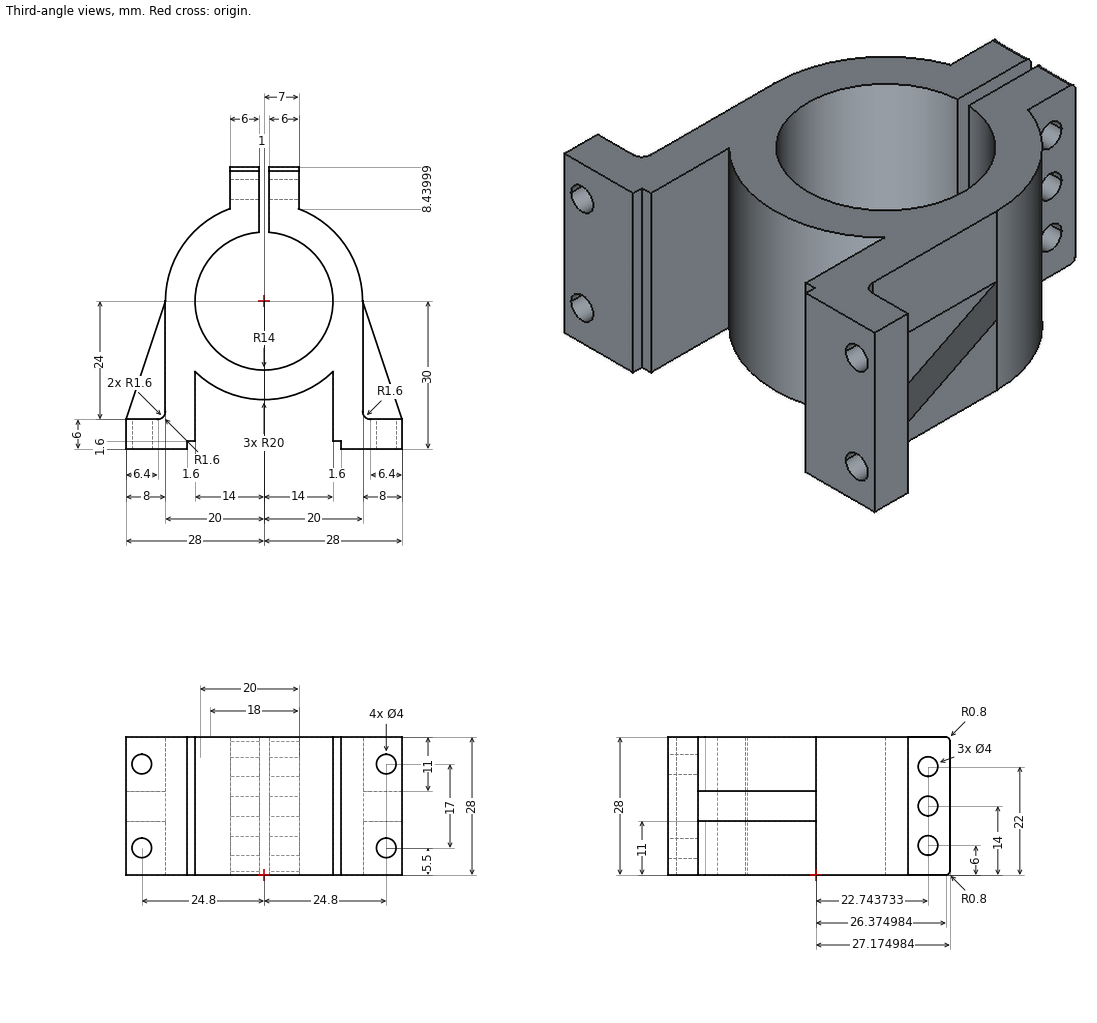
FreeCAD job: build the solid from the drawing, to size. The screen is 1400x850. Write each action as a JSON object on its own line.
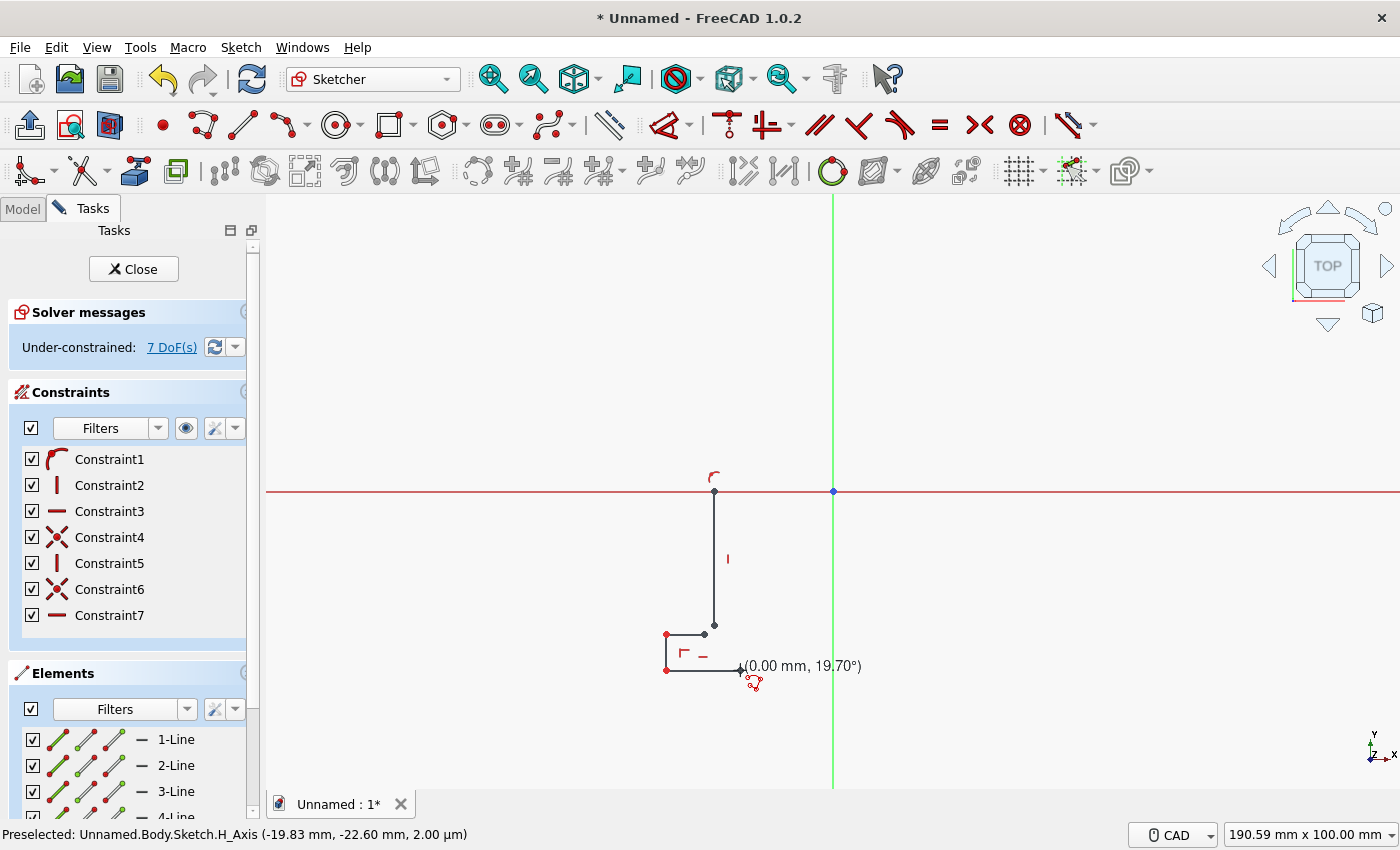
{"action": "scroll", "coordinate": [740, 660], "scroll_direction": "up", "scroll_amount": 3}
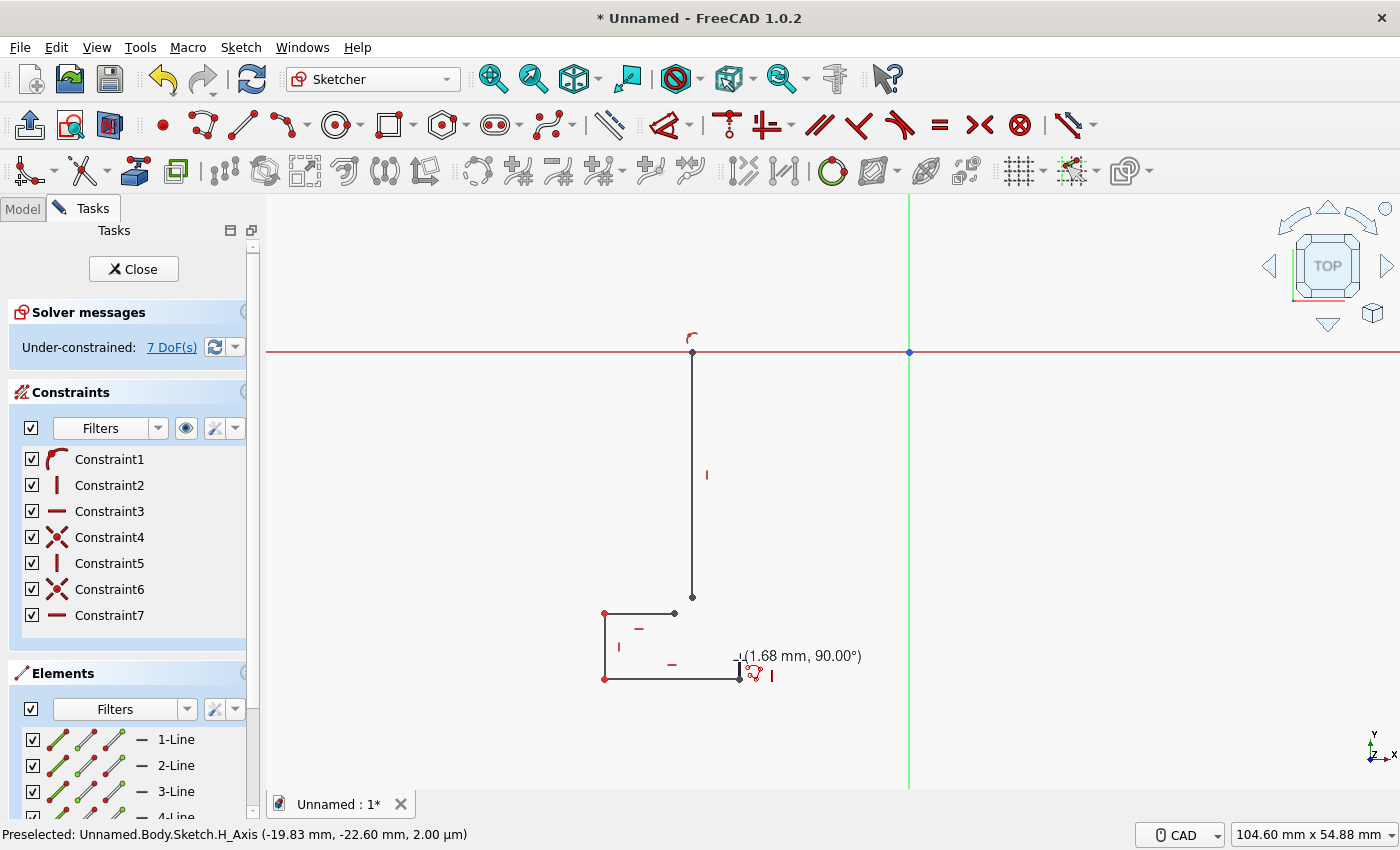
{"action": "left_click", "coordinate": [740, 660]}
{"action": "left_click", "coordinate": [757, 660]}
{"action": "left_click", "coordinate": [757, 507]}
{"action": "right_click", "coordinate": [757, 507]}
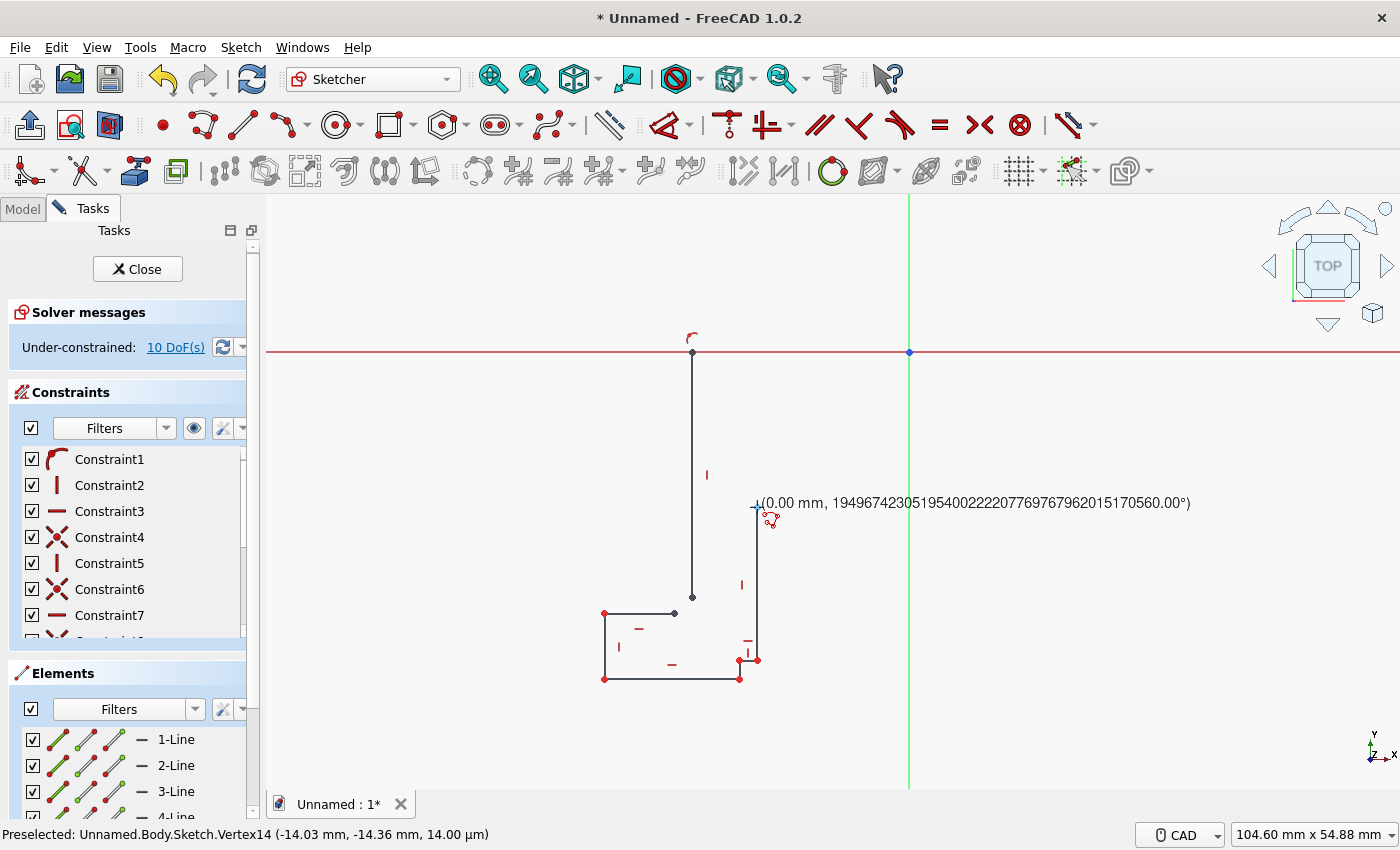
{"action": "left_click", "coordinate": [1061, 507]}
{"action": "left_click", "coordinate": [1061, 660]}
{"action": "left_click", "coordinate": [1078, 660]}
{"action": "left_click", "coordinate": [1078, 678]}
{"action": "left_click", "coordinate": [1213, 678]}
{"action": "left_click", "coordinate": [1213, 613]}
{"action": "left_click", "coordinate": [1143, 613]}
{"action": "right_click", "coordinate": [1143, 613]}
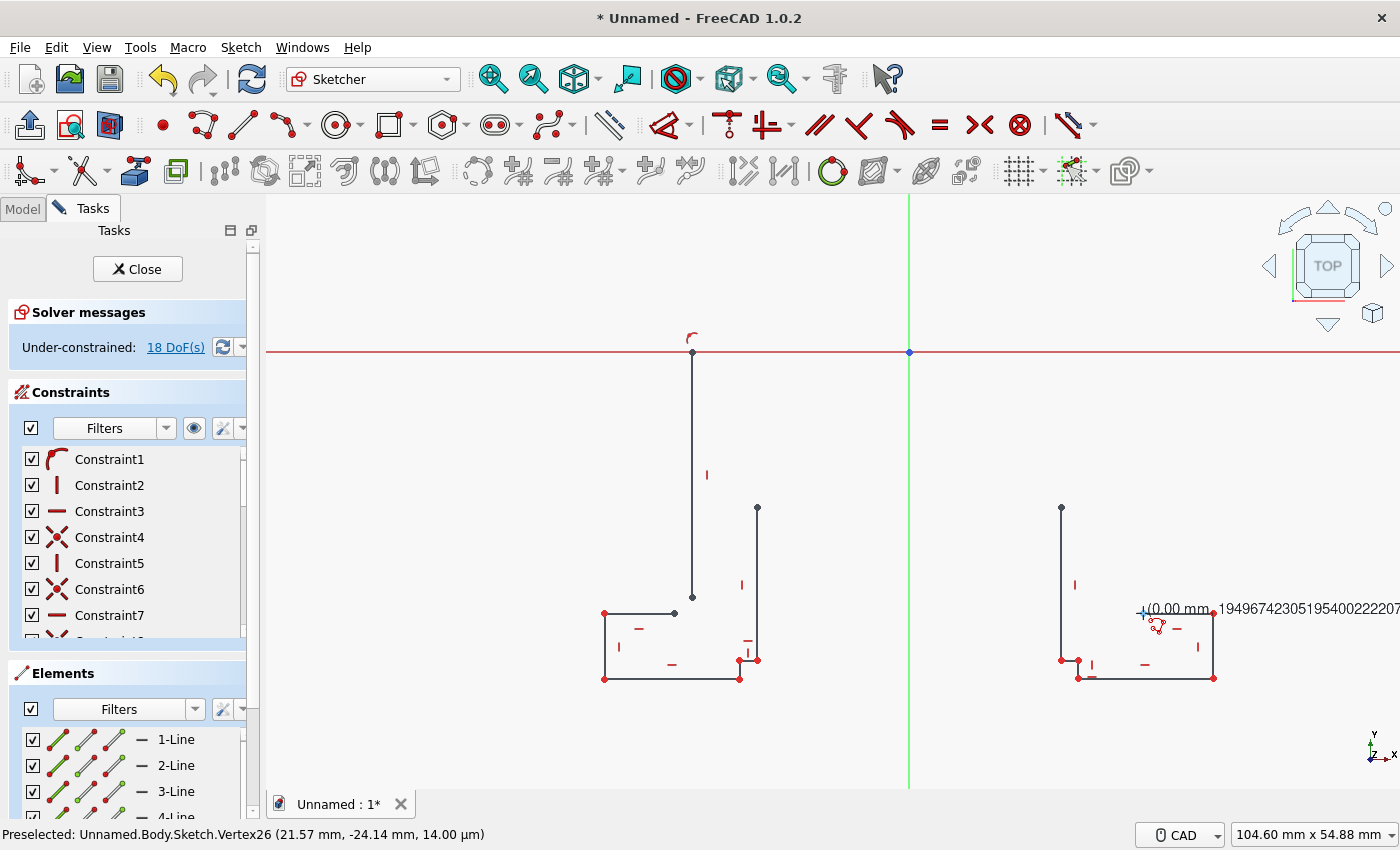
{"action": "left_click", "coordinate": [244, 126]}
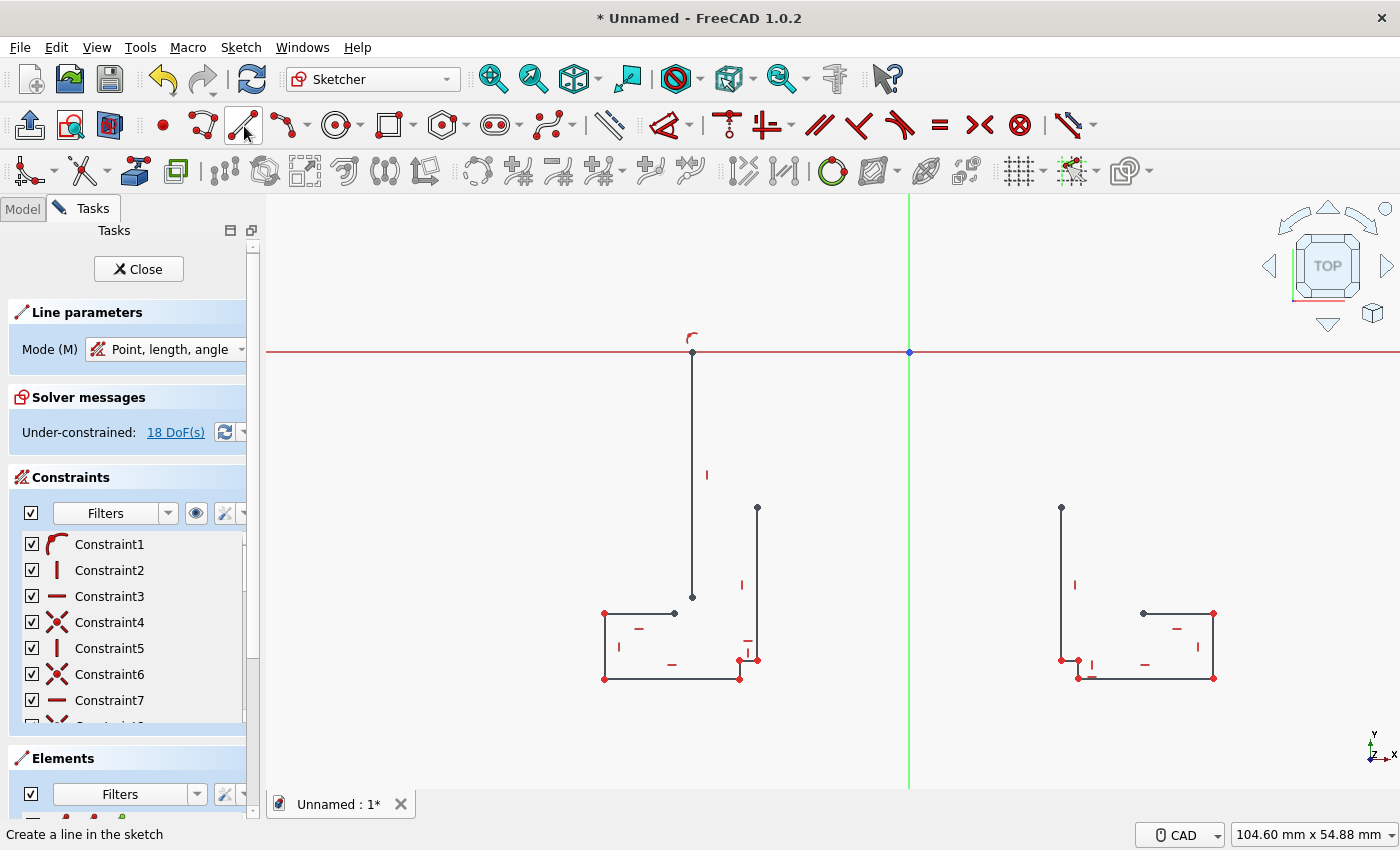
{"action": "left_click", "coordinate": [1126, 595]}
{"action": "left_click", "coordinate": [1126, 352]}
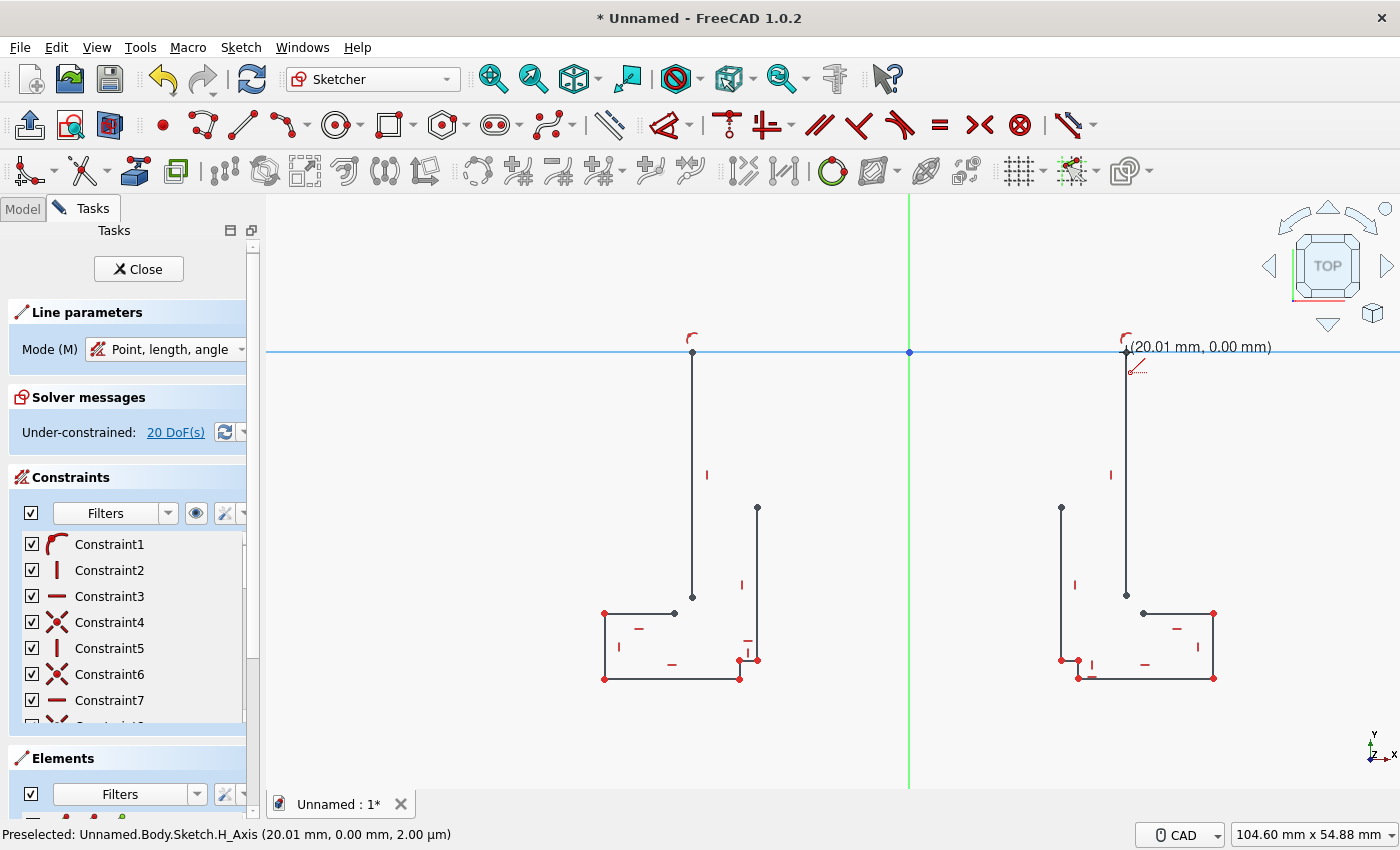
{"action": "left_click", "coordinate": [204, 126]}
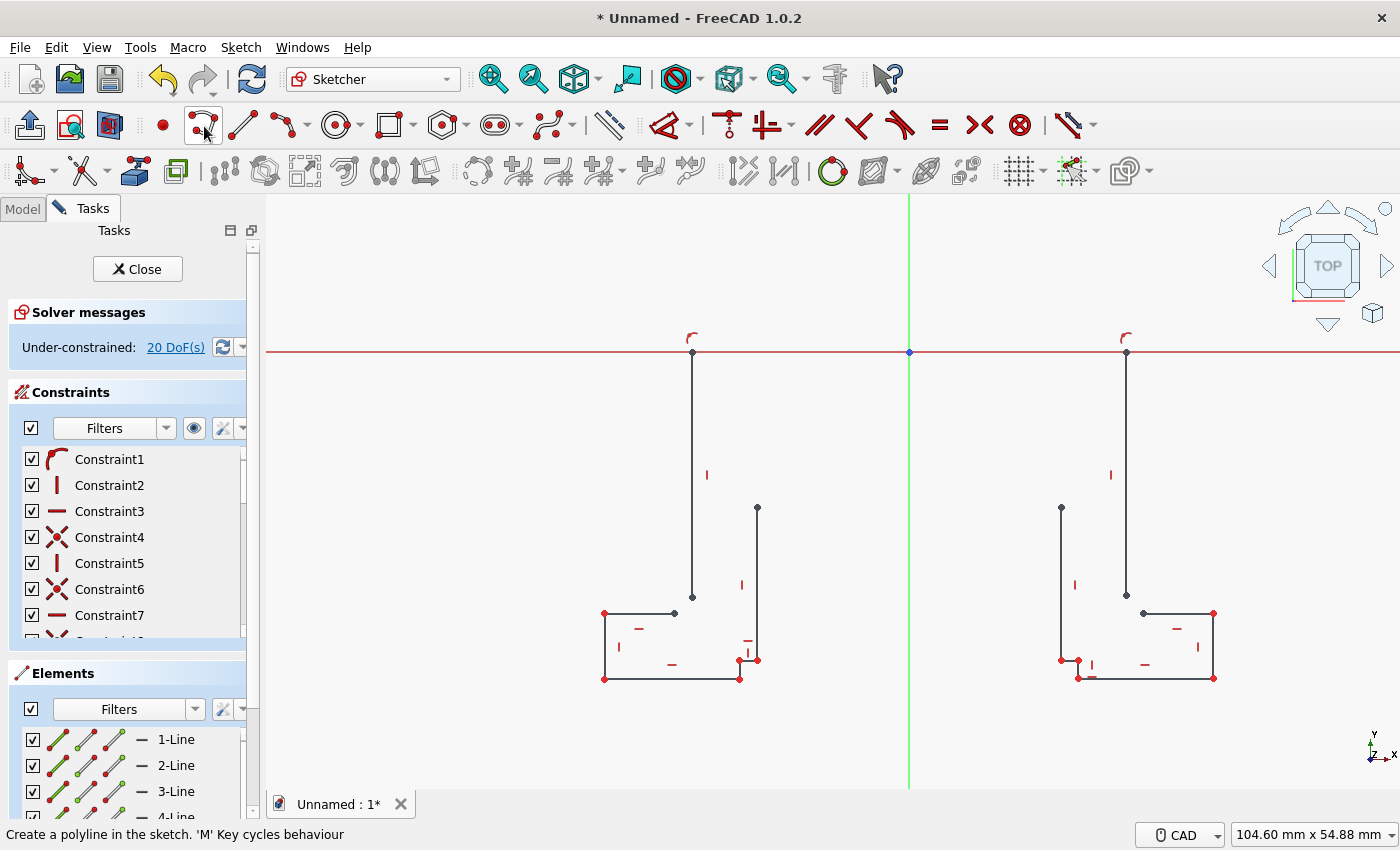
{"action": "scroll", "coordinate": [470, 743], "scroll_direction": "down", "scroll_amount": 2}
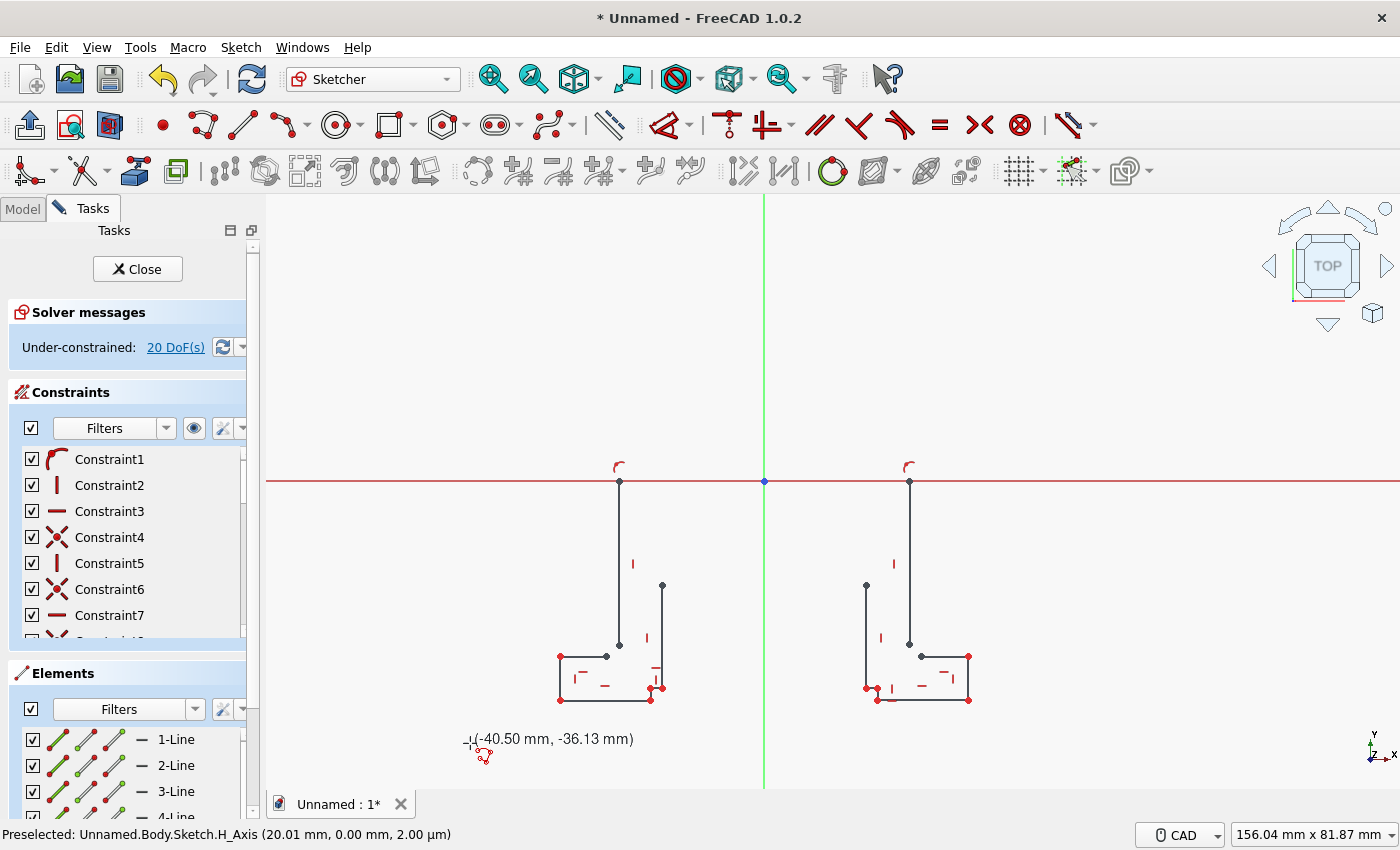
{"action": "left_click", "coordinate": [815, 345]}
{"action": "left_click", "coordinate": [815, 284]}